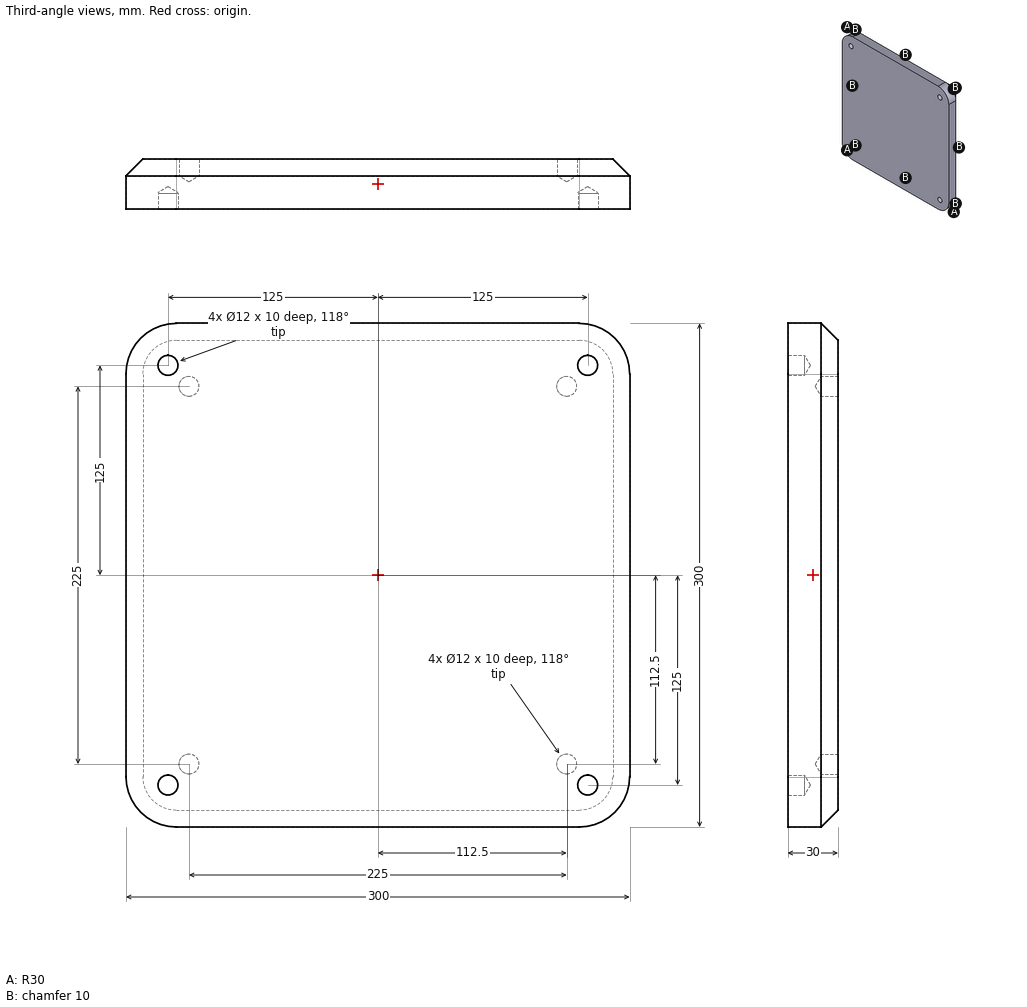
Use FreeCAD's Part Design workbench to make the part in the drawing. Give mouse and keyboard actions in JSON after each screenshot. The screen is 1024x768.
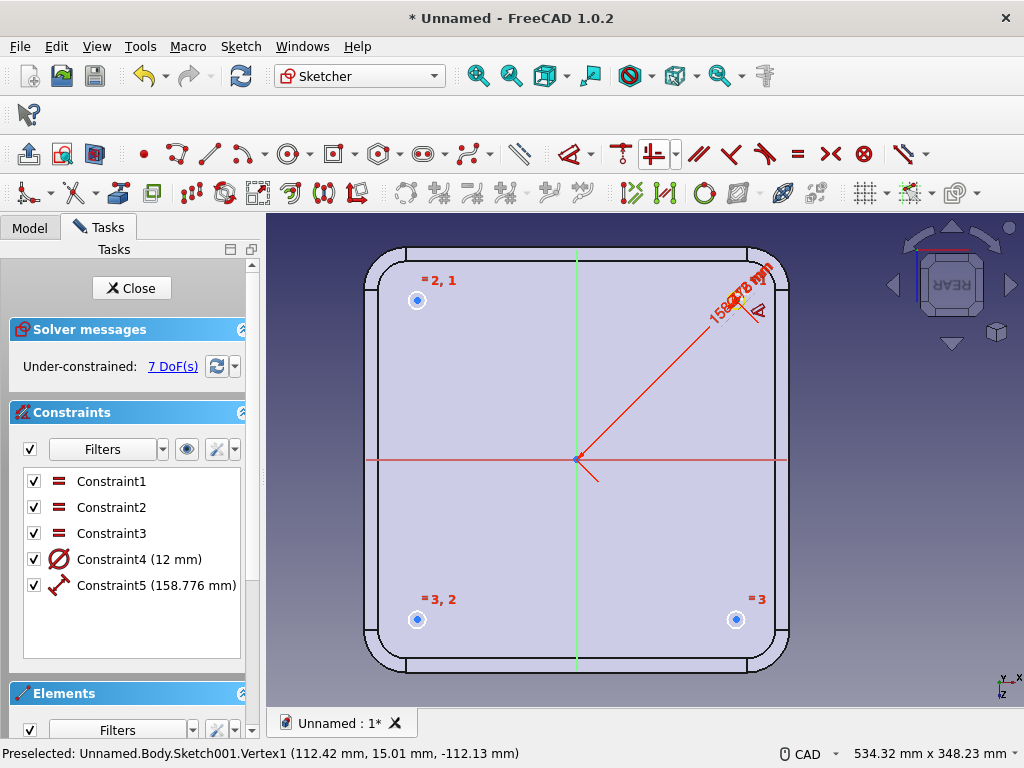
{"action": "left_click", "coordinate": [417, 300]}
{"action": "left_click", "coordinate": [503, 266]}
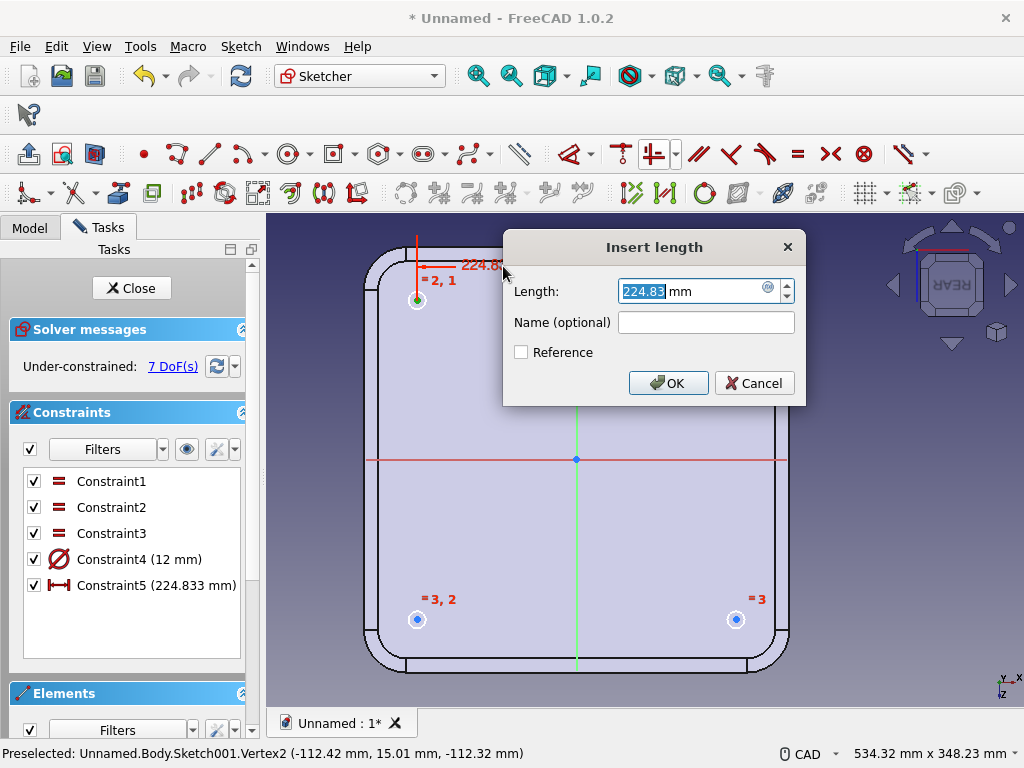
{"action": "type", "text": "225"}
{"action": "key", "text": "Return"}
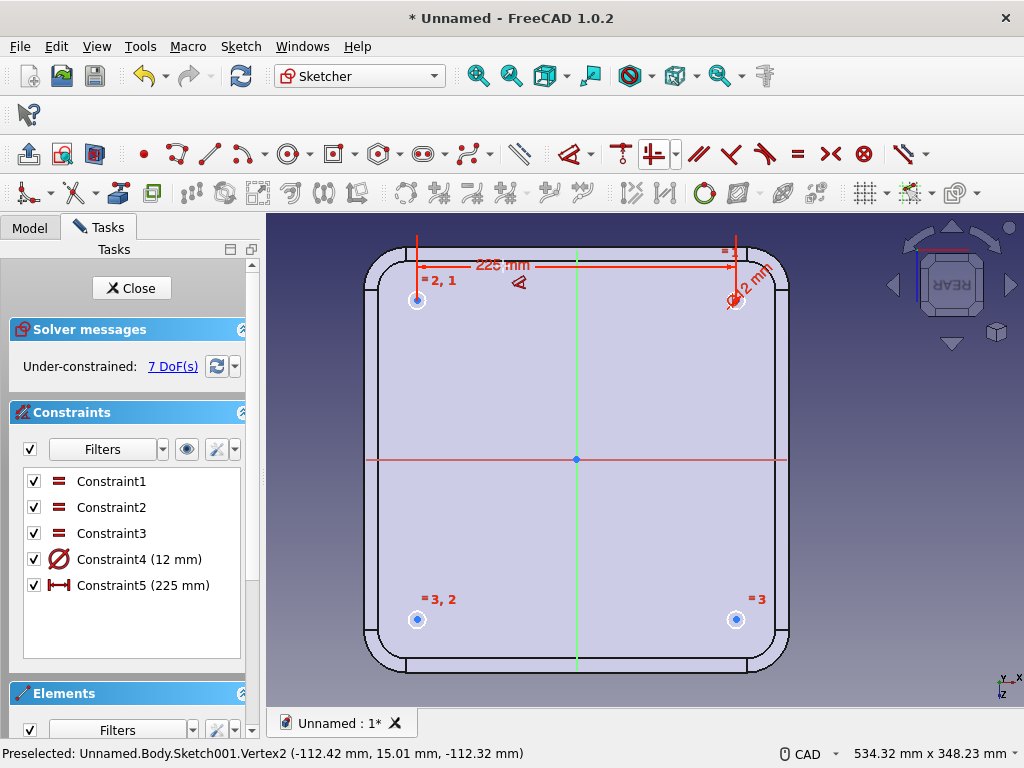
{"action": "left_click", "coordinate": [736, 301]}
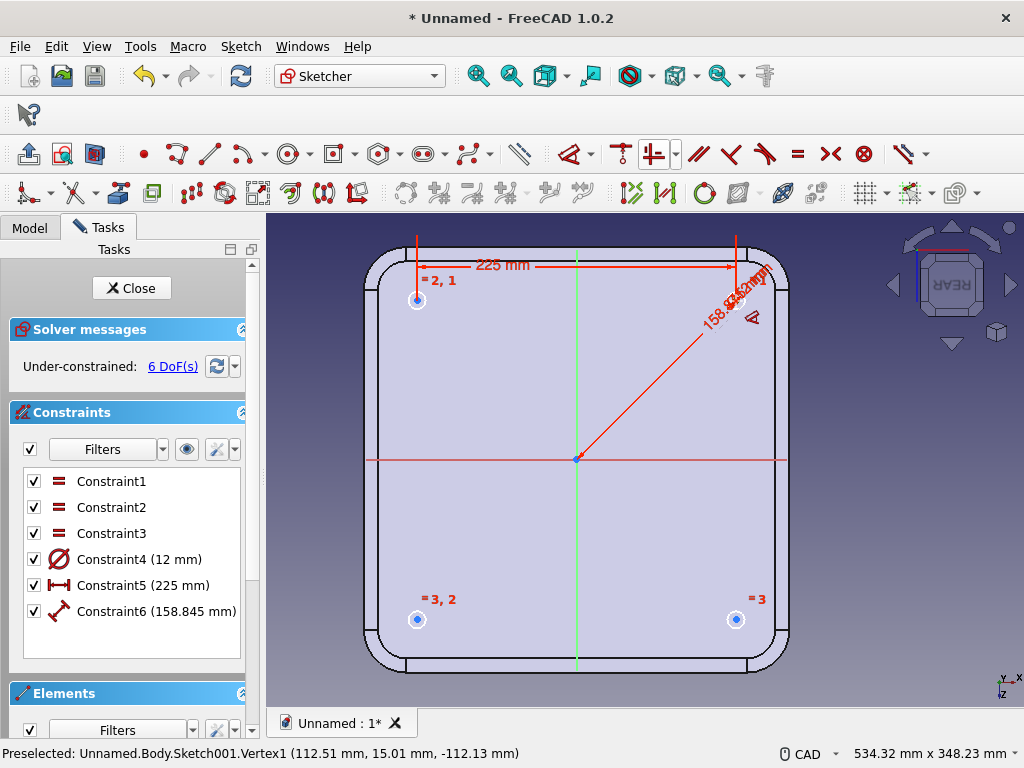
{"action": "left_click", "coordinate": [417, 620]}
{"action": "left_click", "coordinate": [503, 654]}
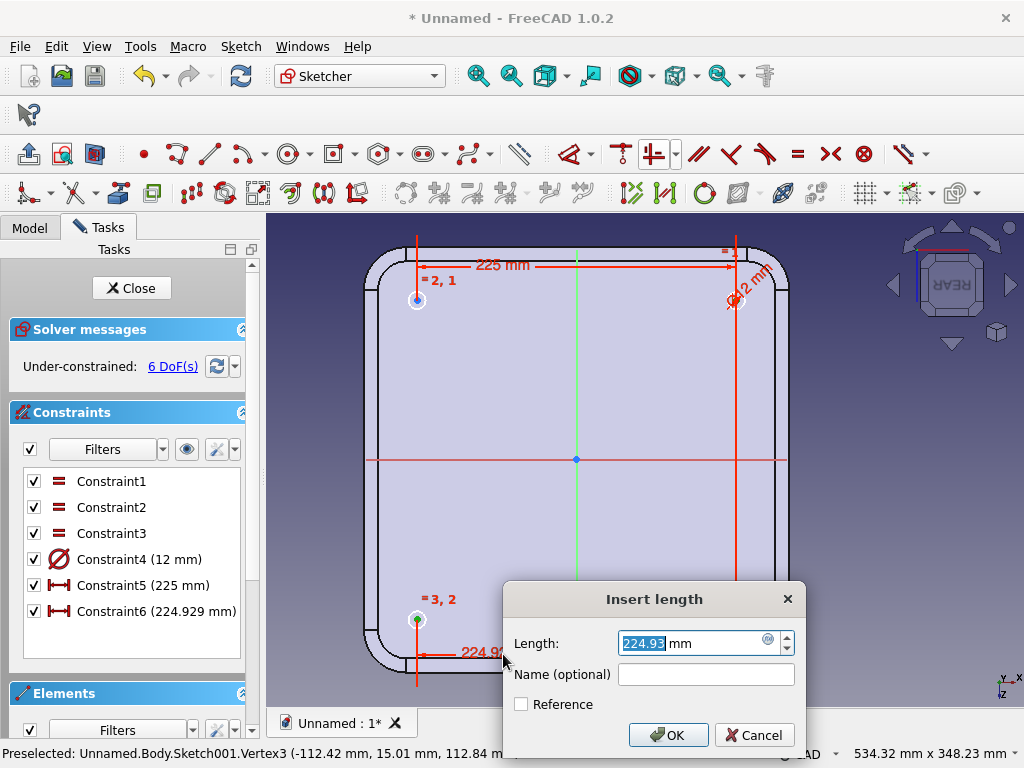
{"action": "type", "text": "225"}
{"action": "key", "text": "Return"}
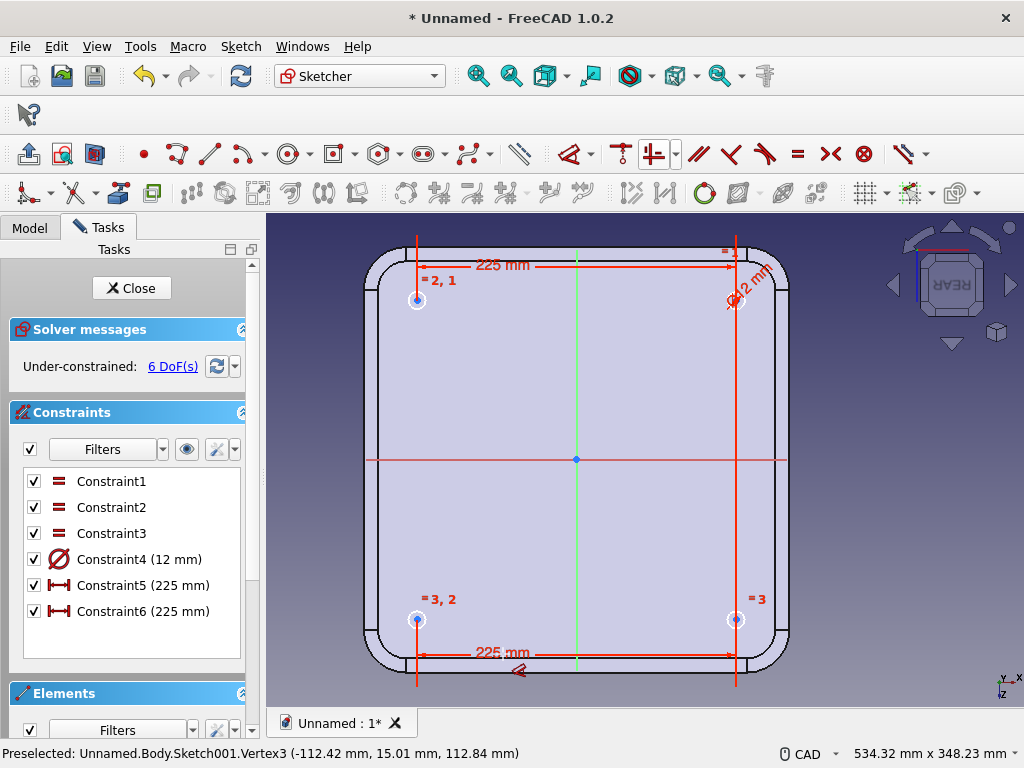
{"action": "left_click", "coordinate": [417, 300]}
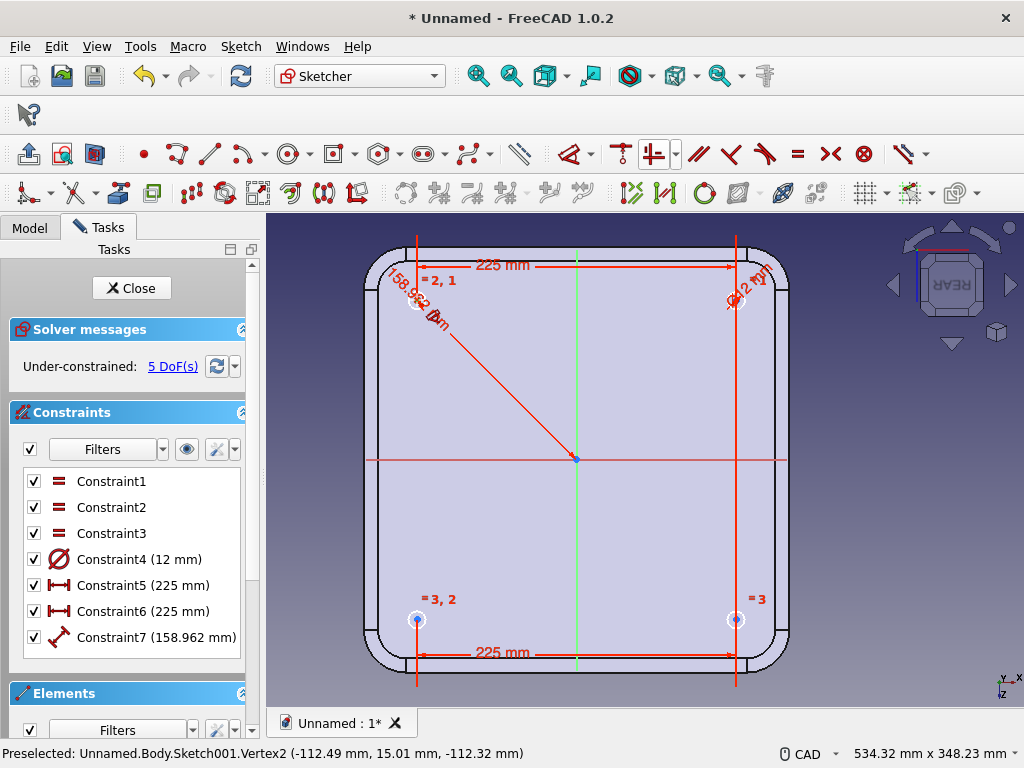
{"action": "left_click", "coordinate": [417, 620]}
{"action": "left_click", "coordinate": [383, 387]}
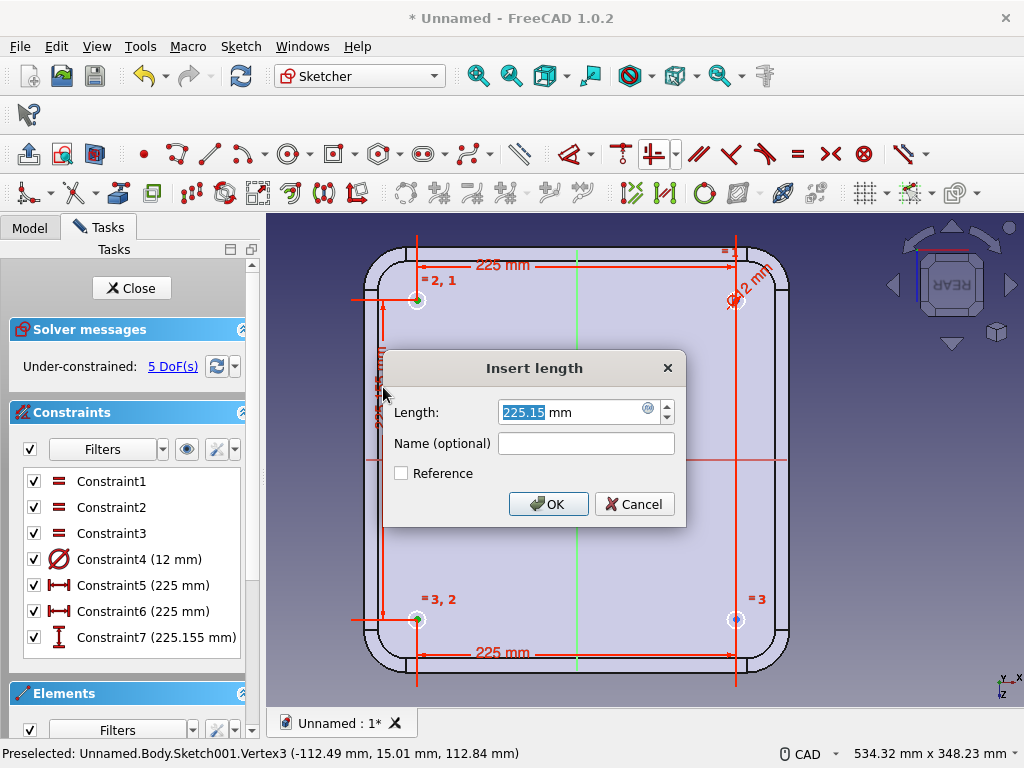
{"action": "type", "text": "225"}
{"action": "key", "text": "Return"}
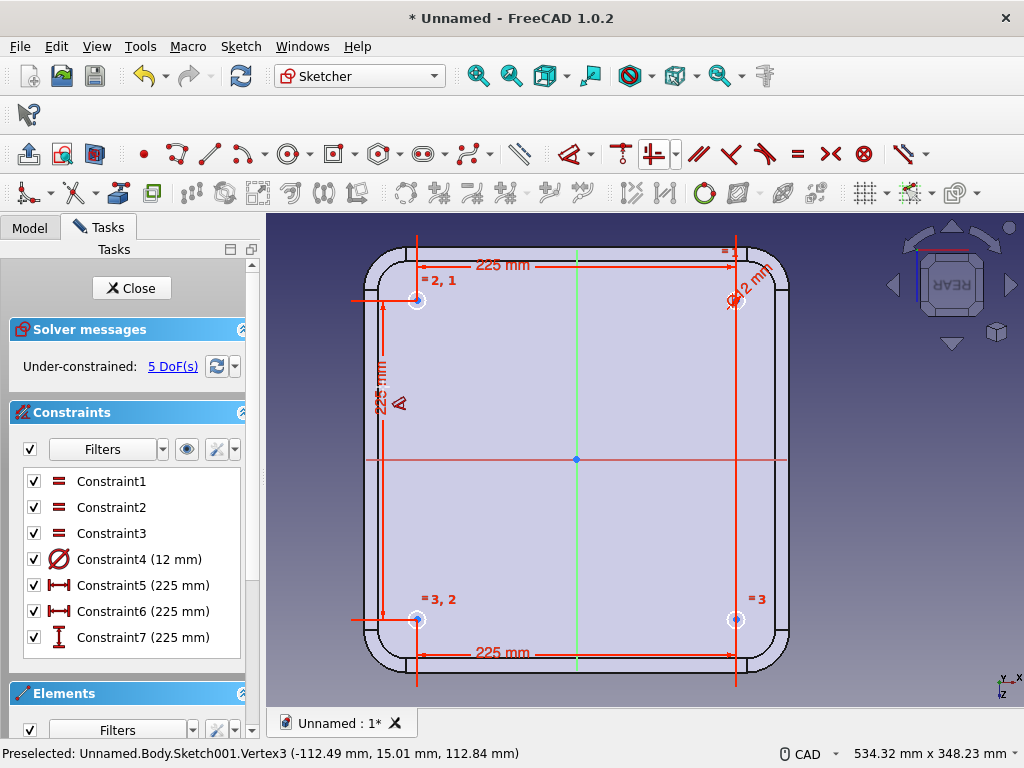
{"action": "left_click", "coordinate": [736, 301]}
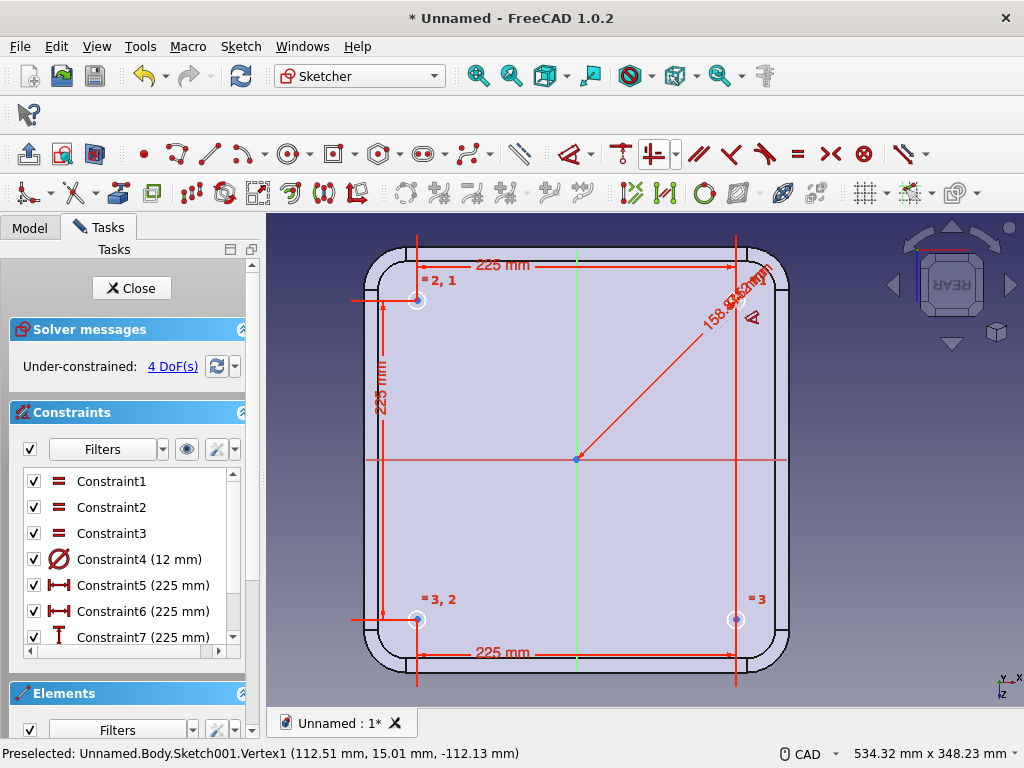
{"action": "left_click", "coordinate": [417, 620]}
{"action": "left_click", "coordinate": [770, 387]}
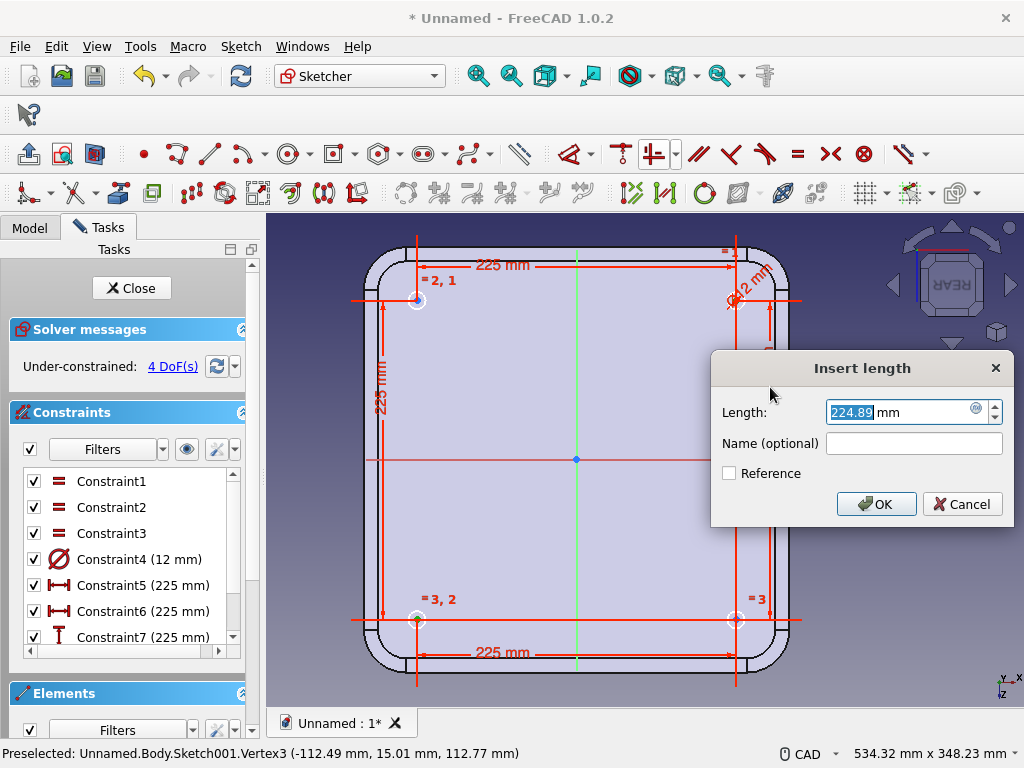
{"action": "type", "text": "225"}
{"action": "key", "text": "Return"}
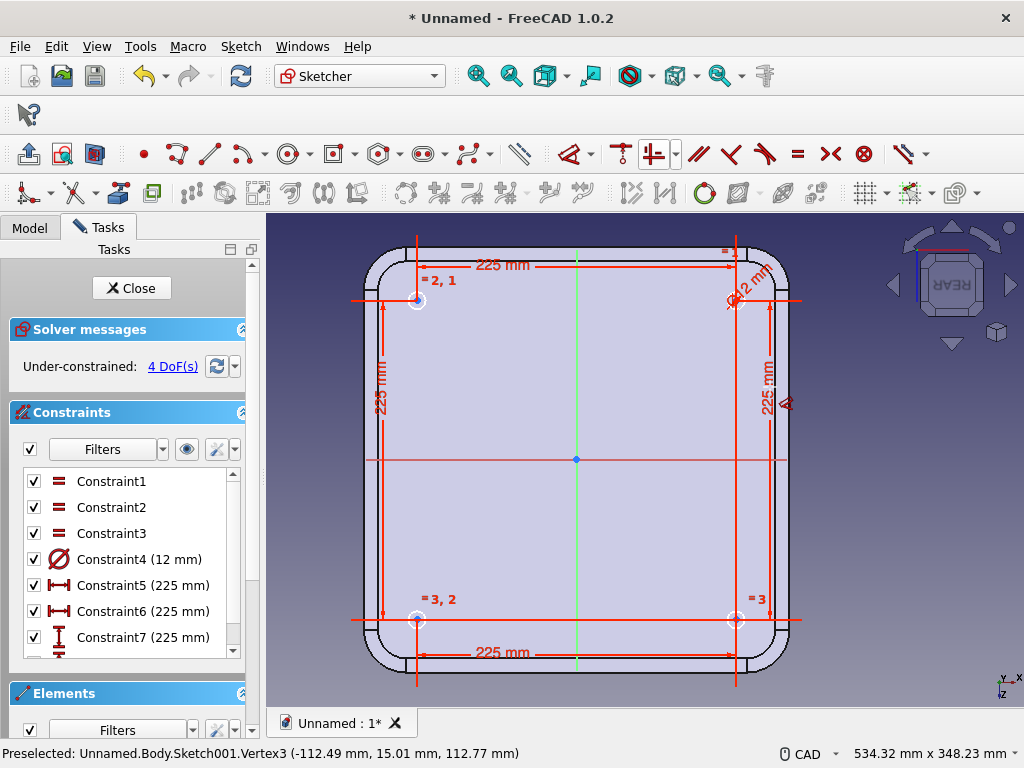
{"action": "left_click", "coordinate": [417, 620]}